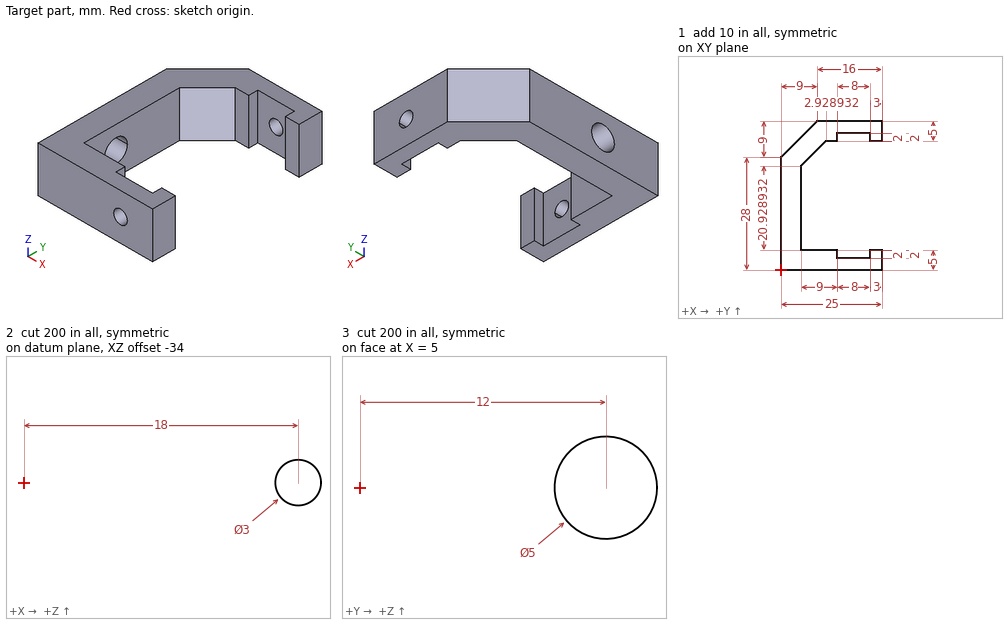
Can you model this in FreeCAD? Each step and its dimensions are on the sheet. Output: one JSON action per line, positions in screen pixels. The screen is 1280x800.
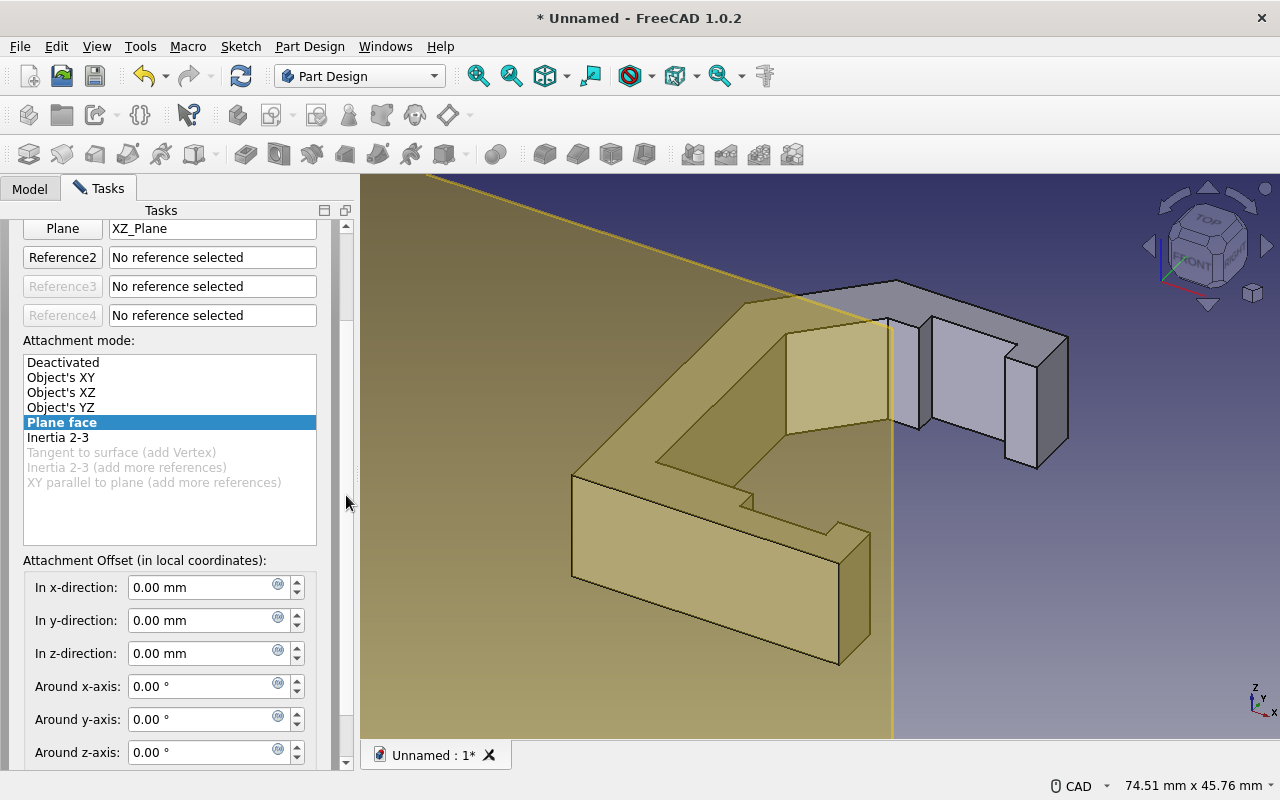
{"action": "triple_click", "coordinate": [210, 654]}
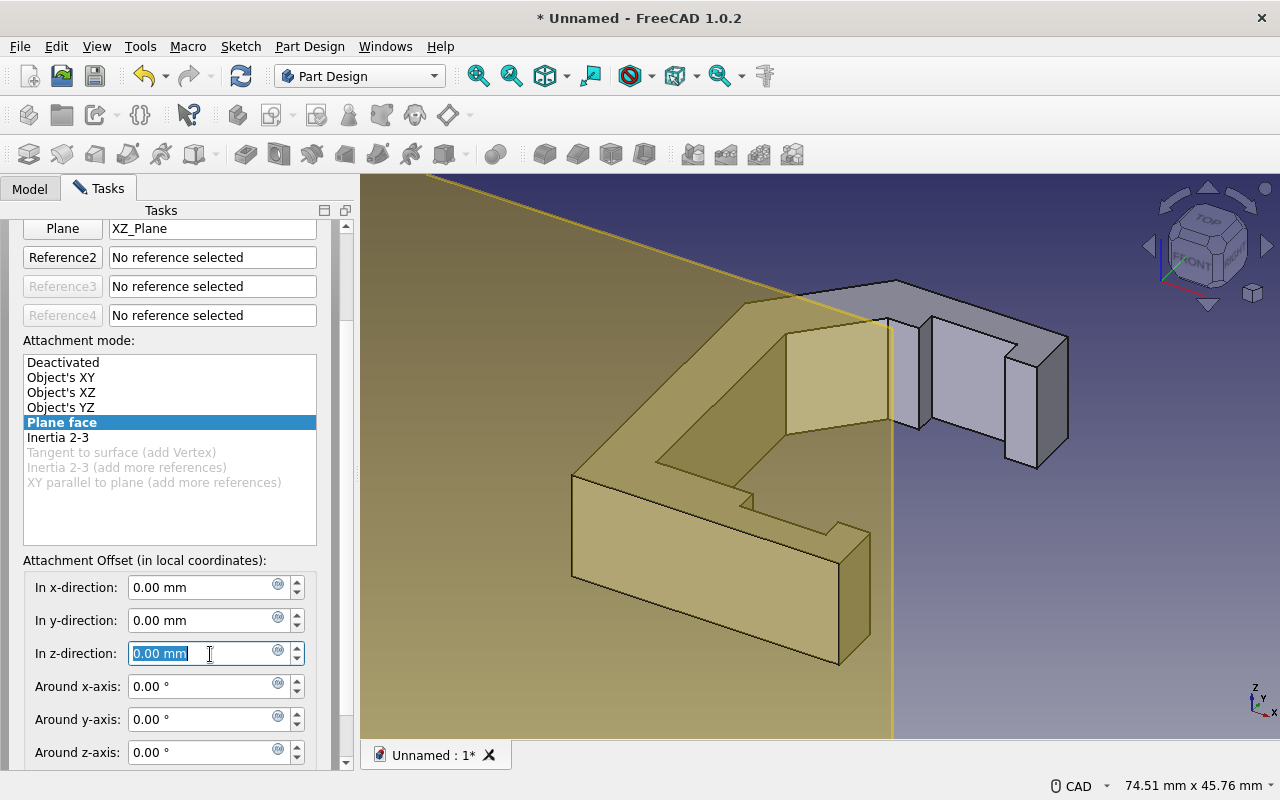
{"action": "type", "text": "-34"}
{"action": "key", "text": "Tab"}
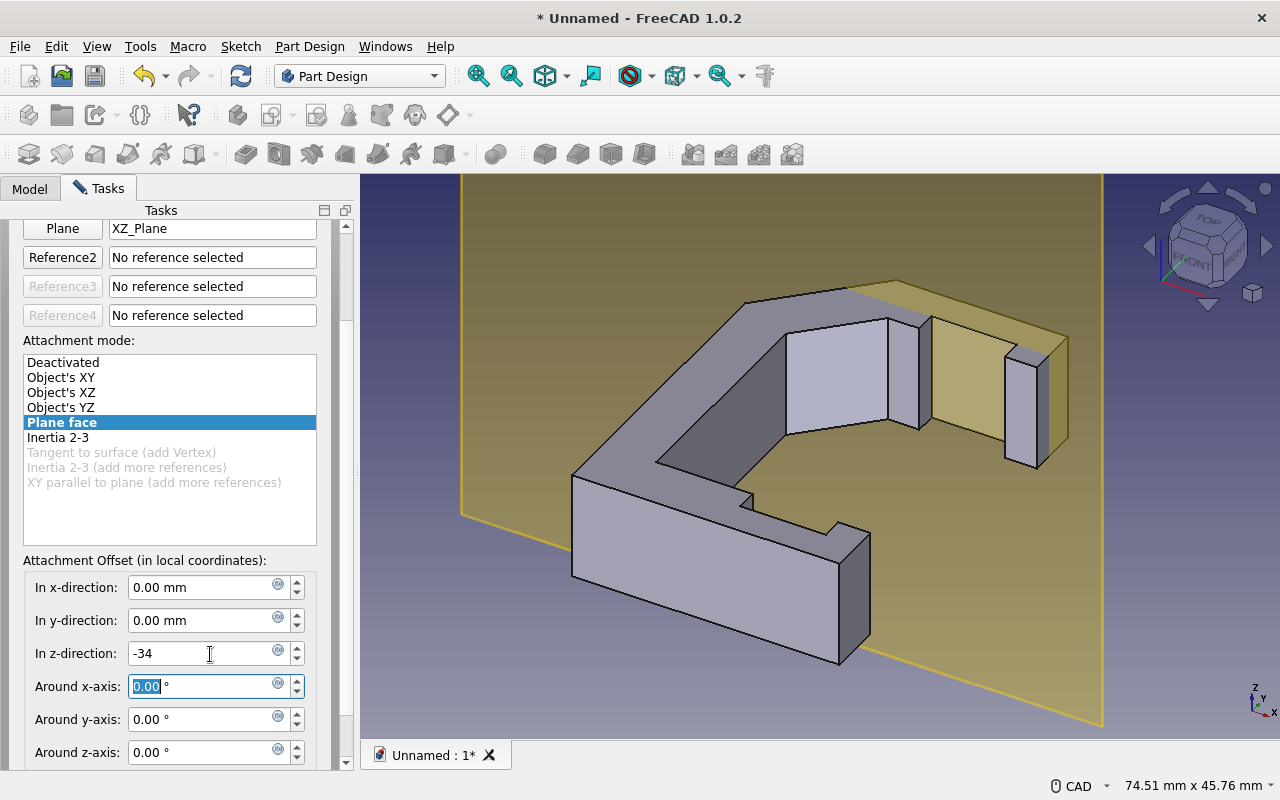
{"action": "scroll", "coordinate": [346, 495], "scroll_direction": "up", "scroll_amount": 3}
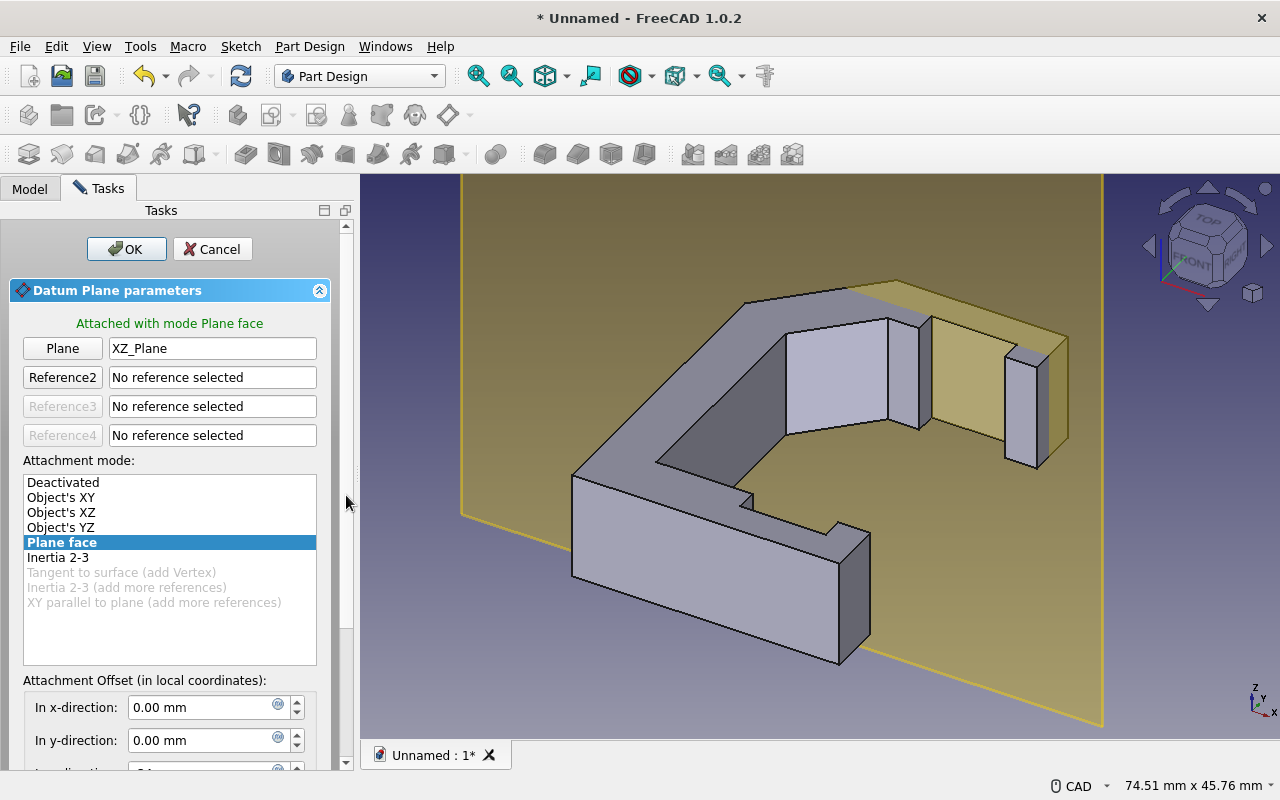
{"action": "left_click", "coordinate": [127, 249]}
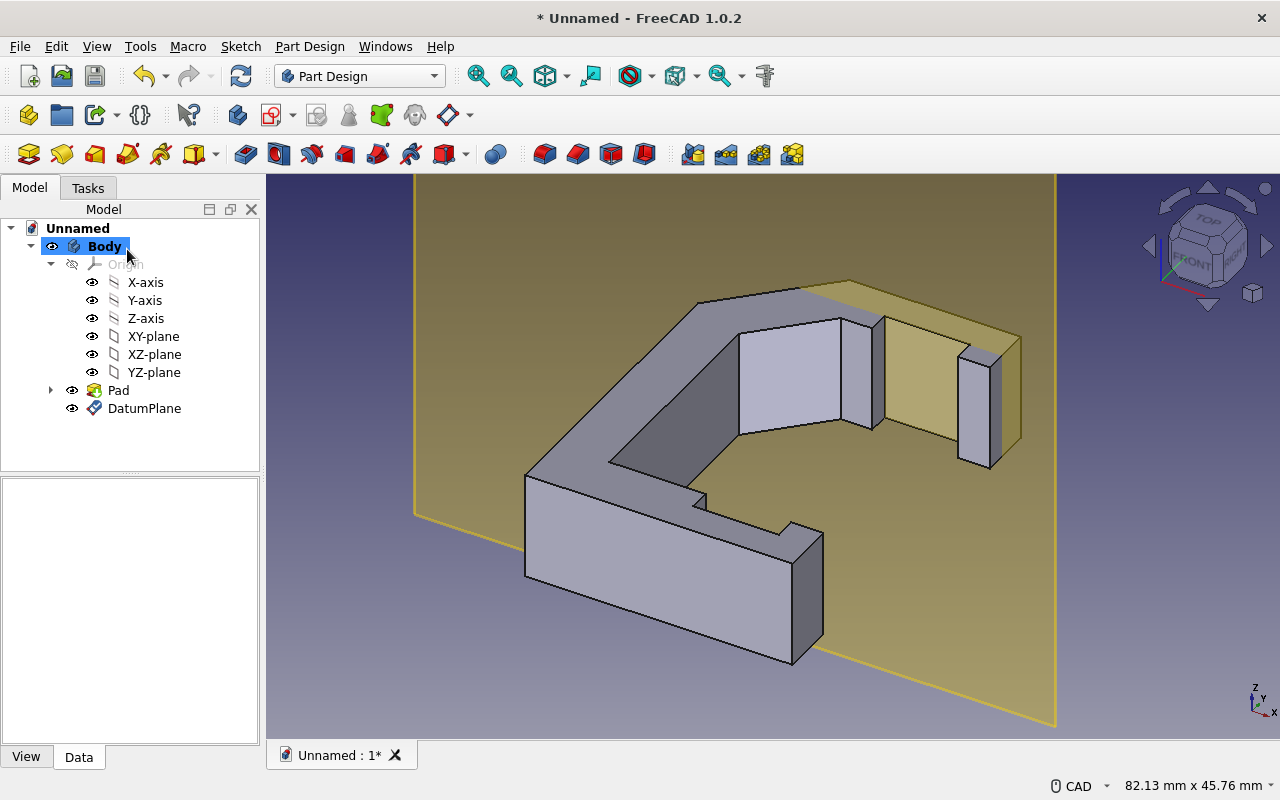
{"action": "left_click", "coordinate": [117, 408]}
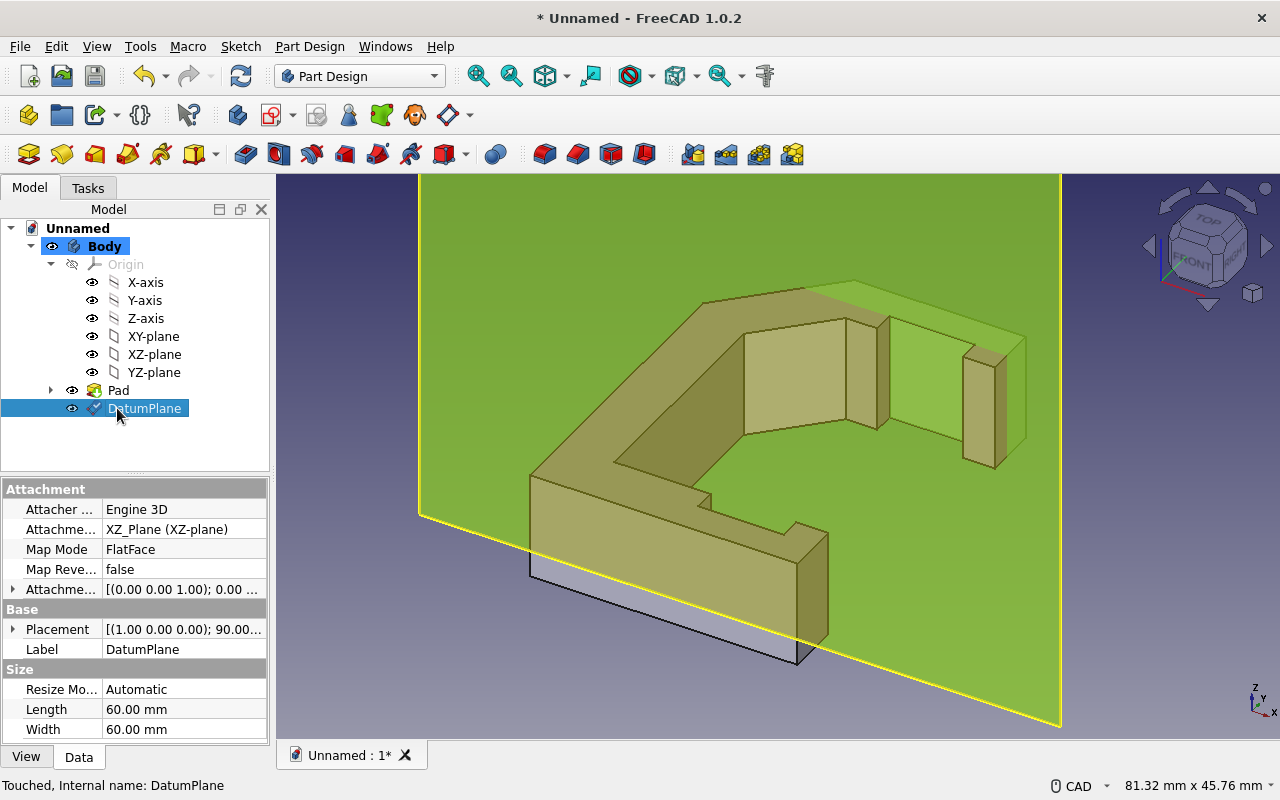
{"action": "left_click", "coordinate": [270, 116]}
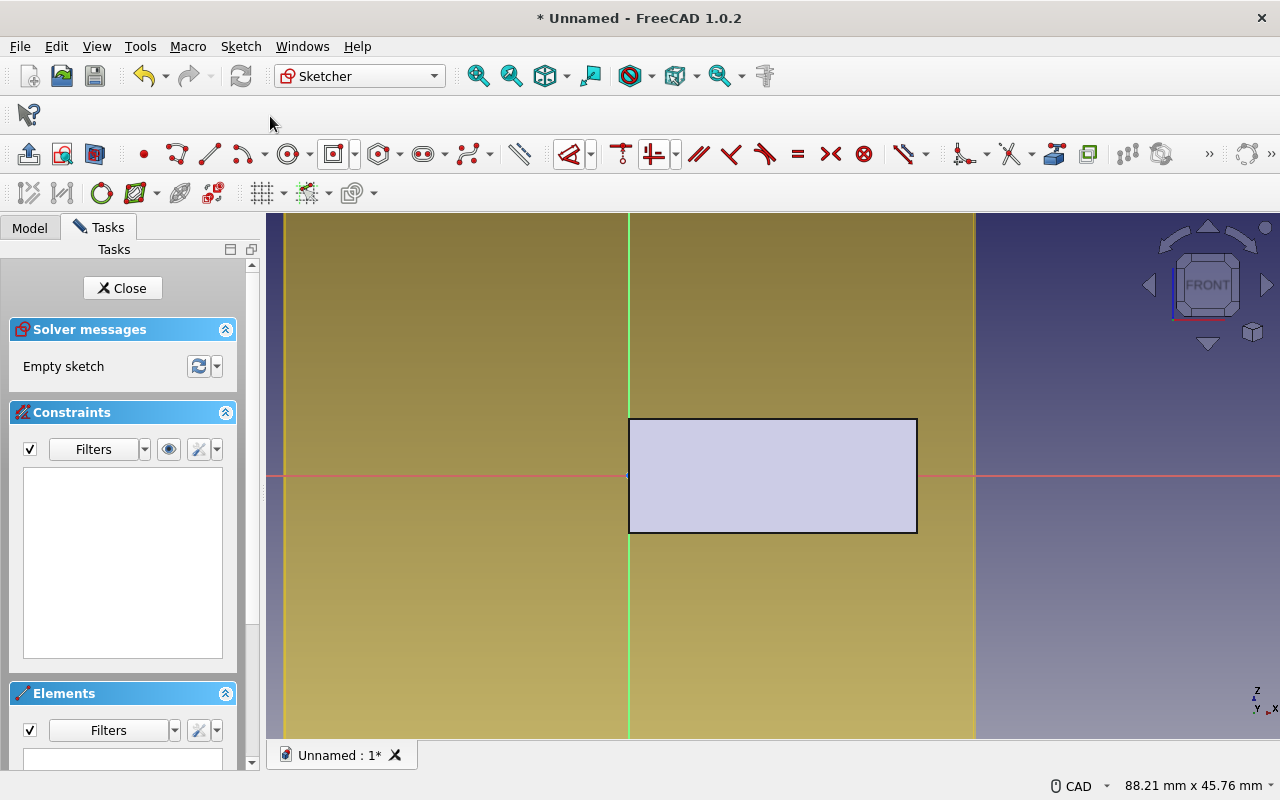
{"action": "left_click", "coordinate": [95, 154]}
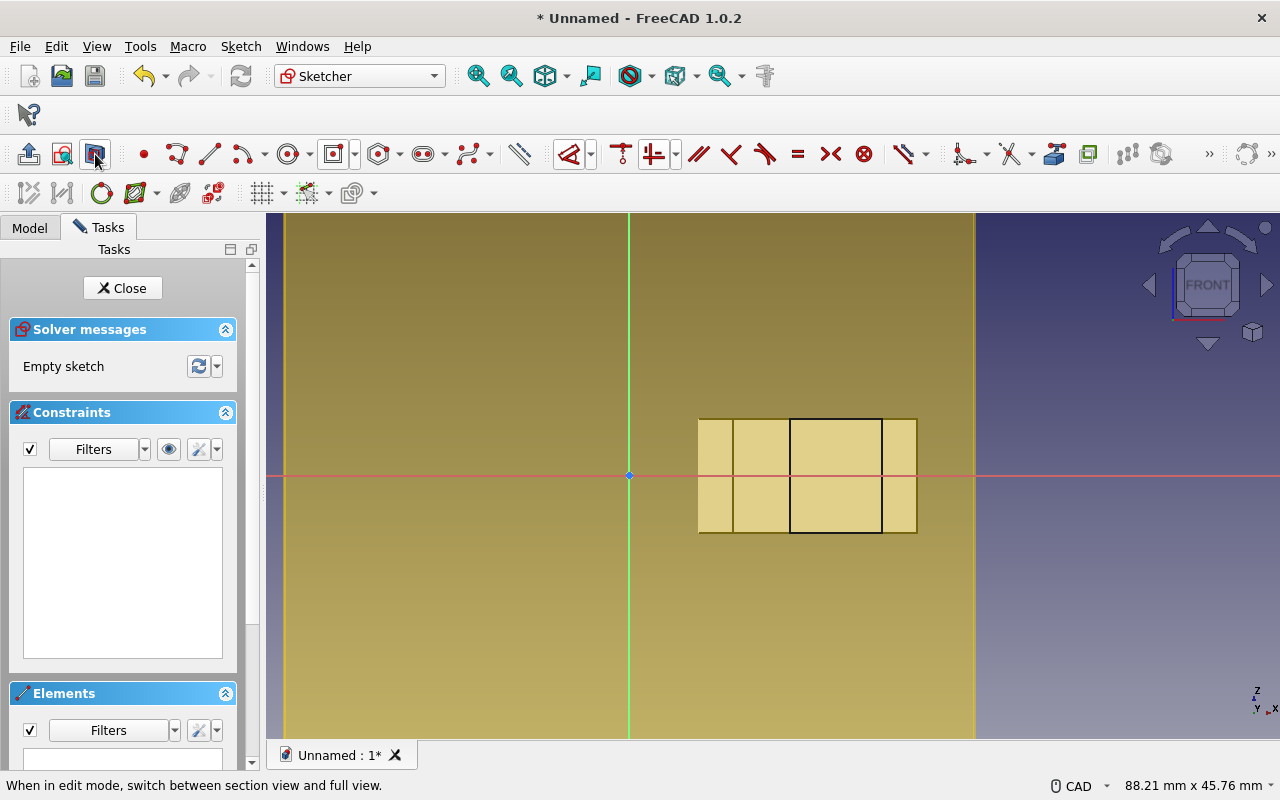
{"action": "scroll", "coordinate": [853, 476], "scroll_direction": "up", "scroll_amount": 11}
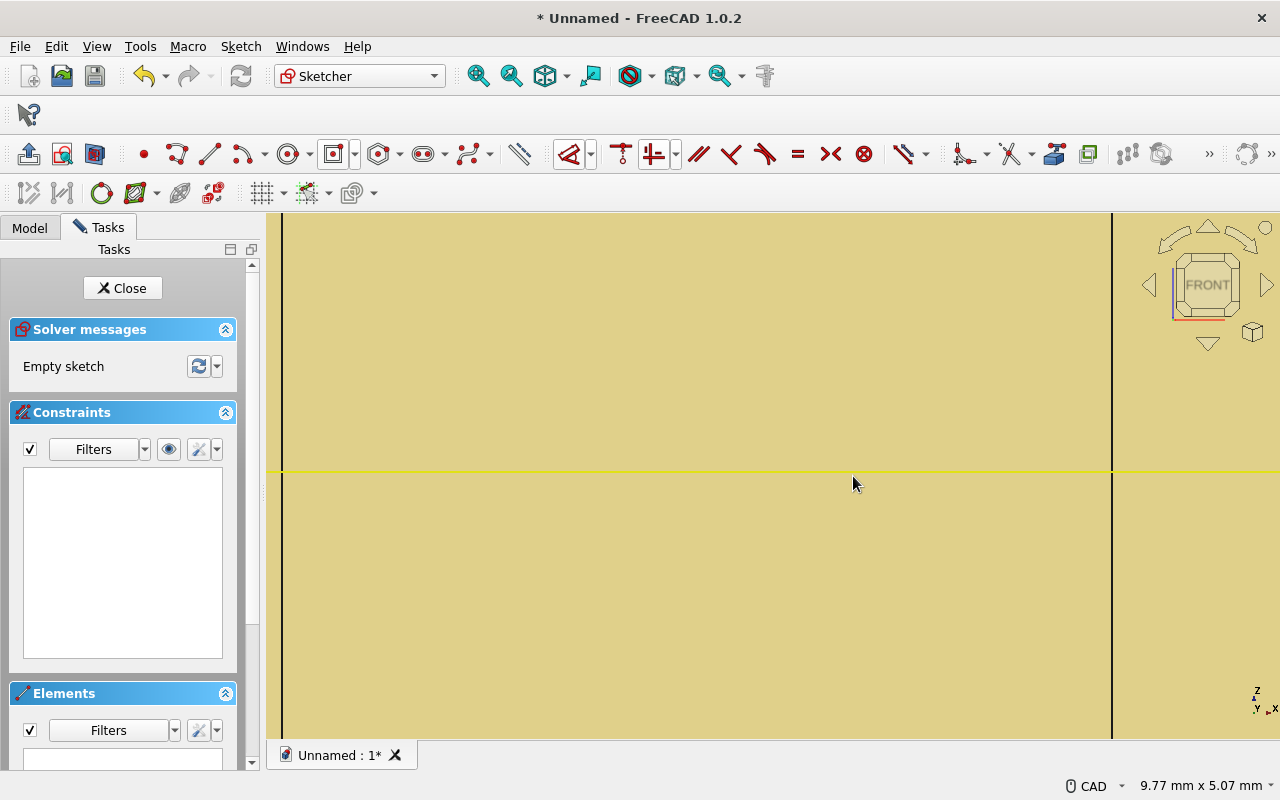
{"action": "key", "text": "g c"}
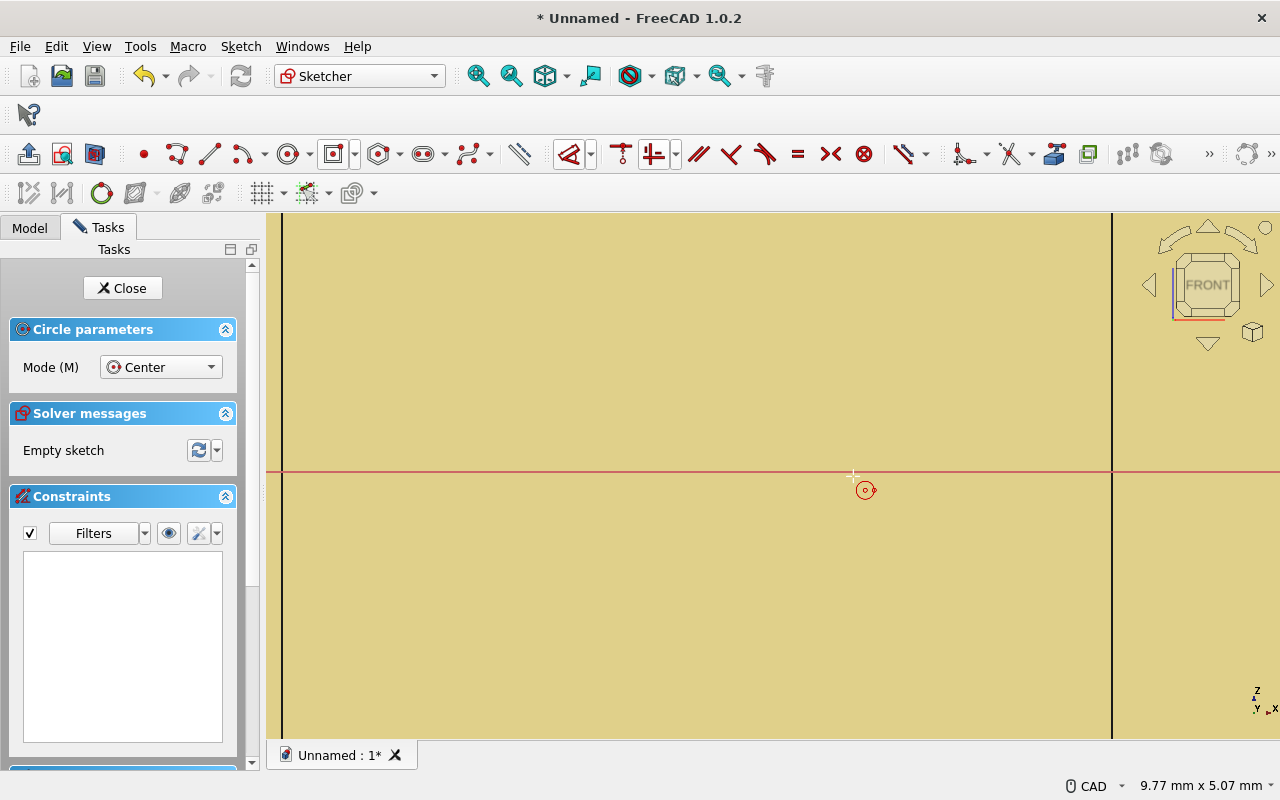
{"action": "left_click", "coordinate": [697, 472]}
{"action": "left_click", "coordinate": [807, 362]}
{"action": "key", "text": "Escape"}